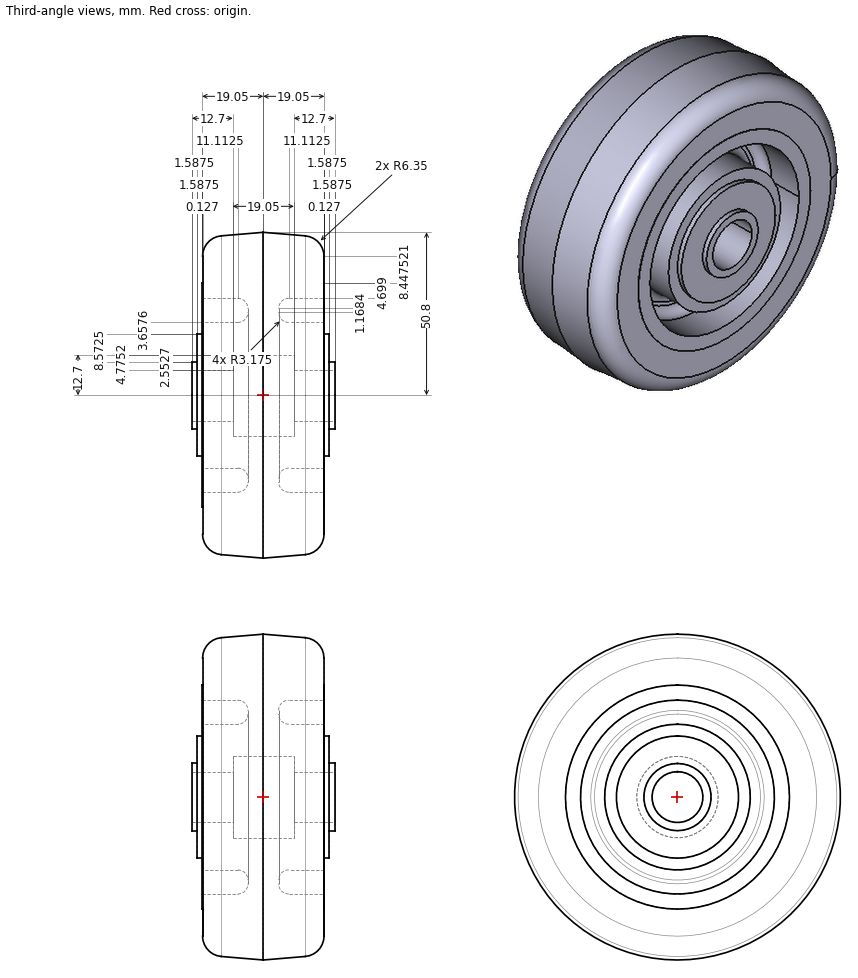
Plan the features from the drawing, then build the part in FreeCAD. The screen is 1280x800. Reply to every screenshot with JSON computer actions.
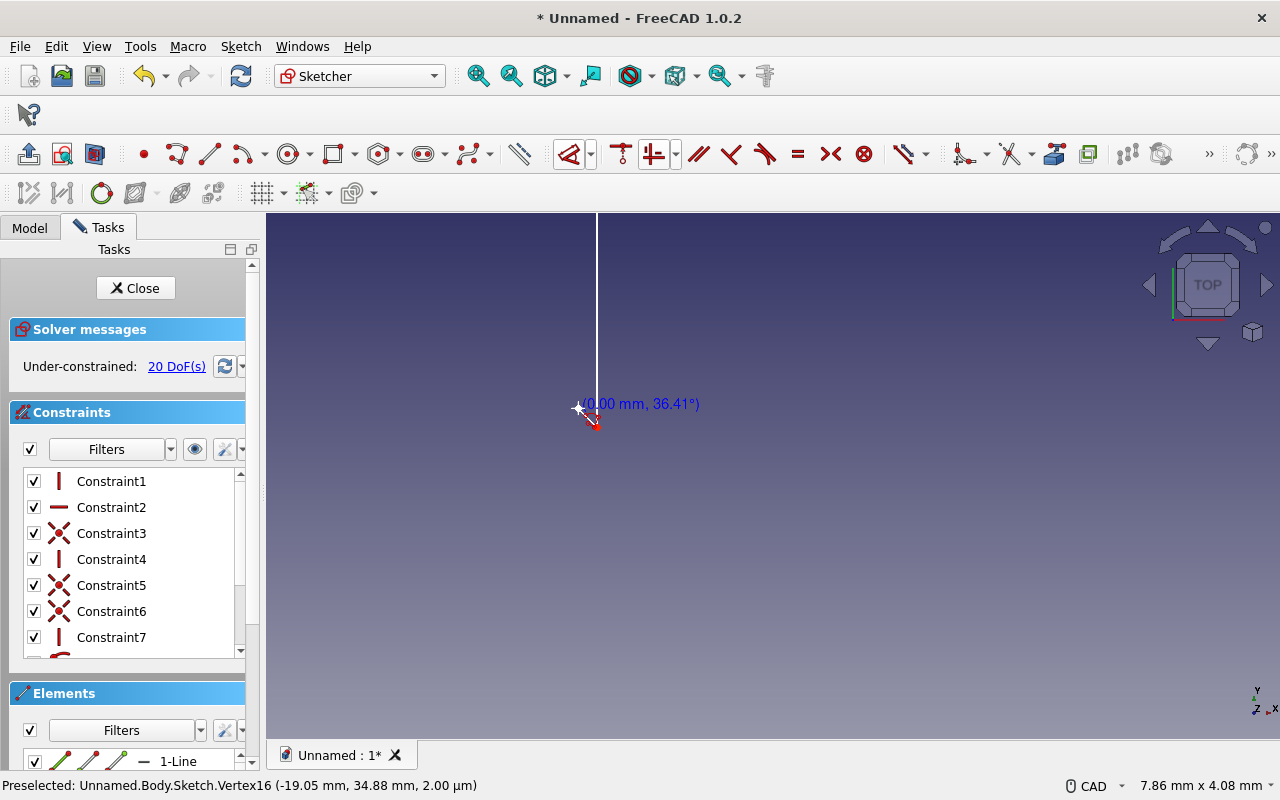
{"action": "scroll", "coordinate": [582, 415], "scroll_direction": "down", "scroll_amount": 15}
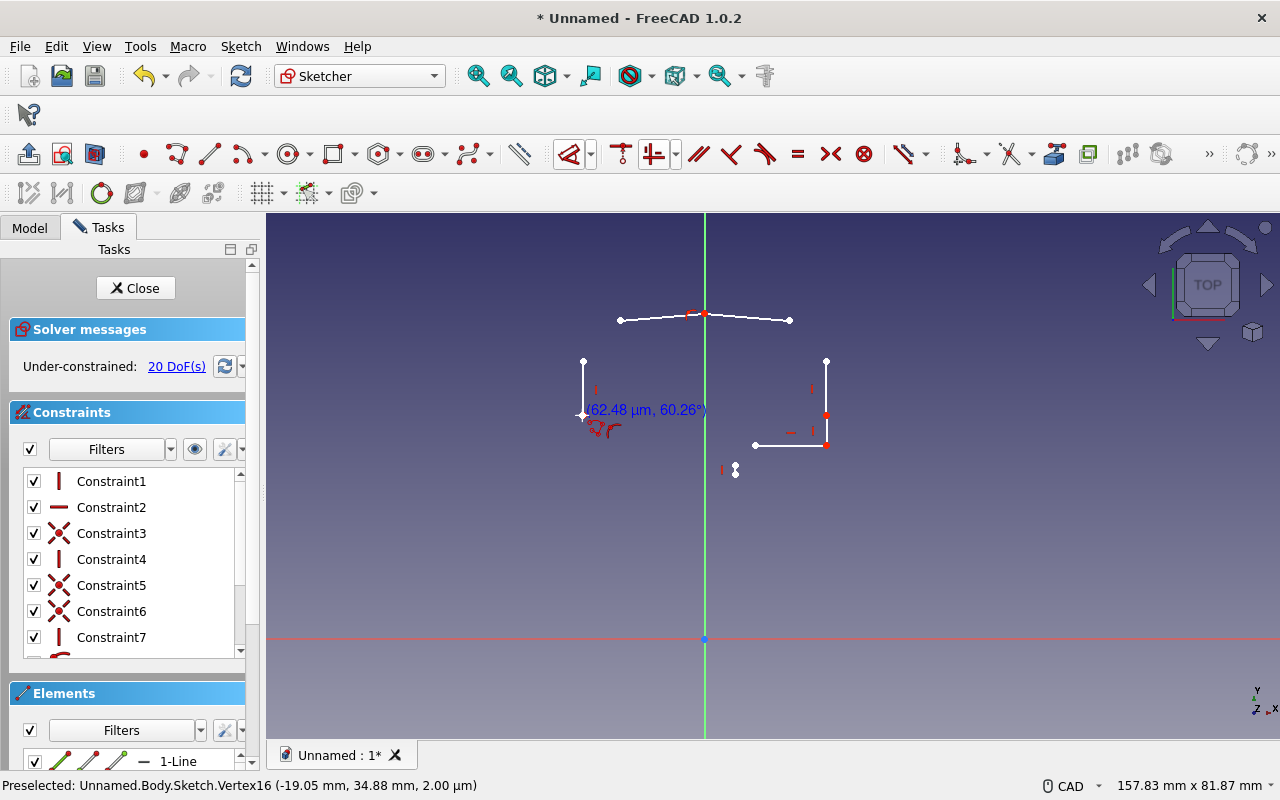
{"action": "left_click", "coordinate": [582, 445]}
{"action": "left_click", "coordinate": [654, 445]}
{"action": "right_click", "coordinate": [654, 445]}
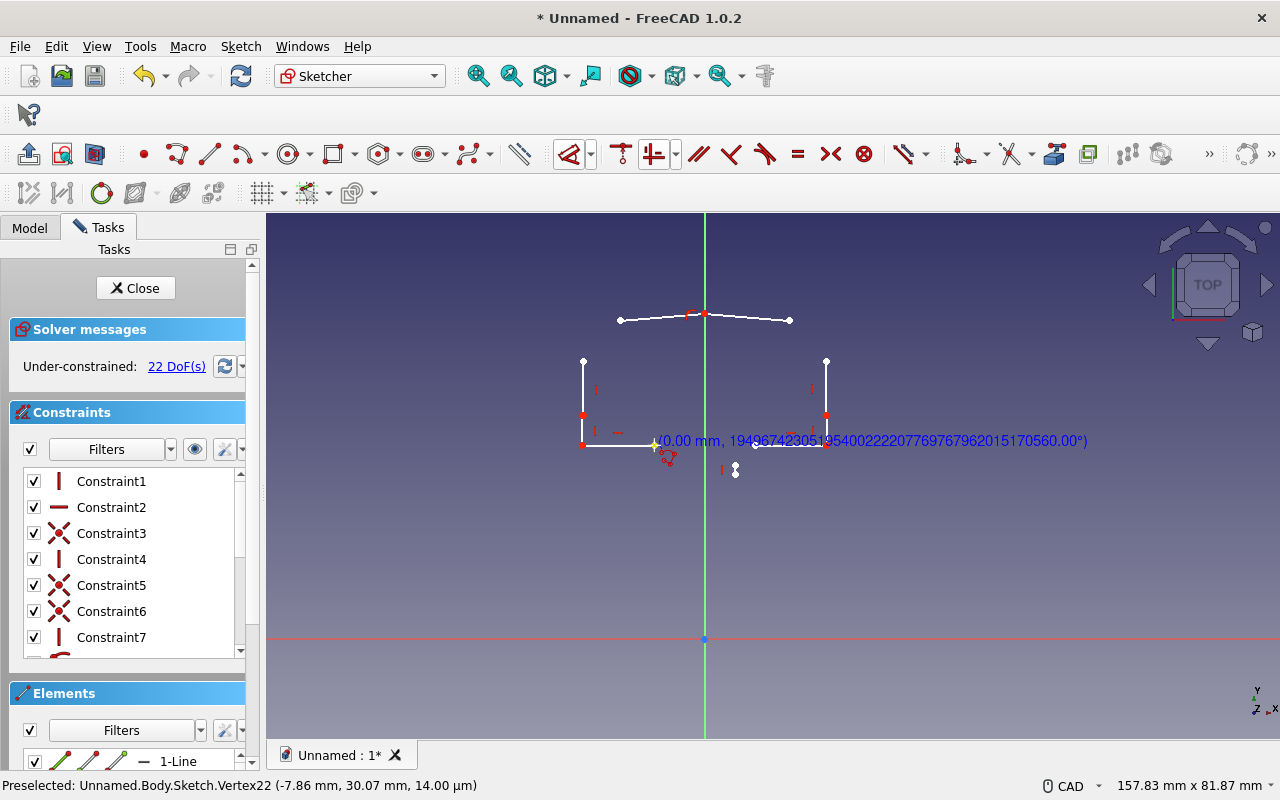
{"action": "left_click", "coordinate": [210, 154]}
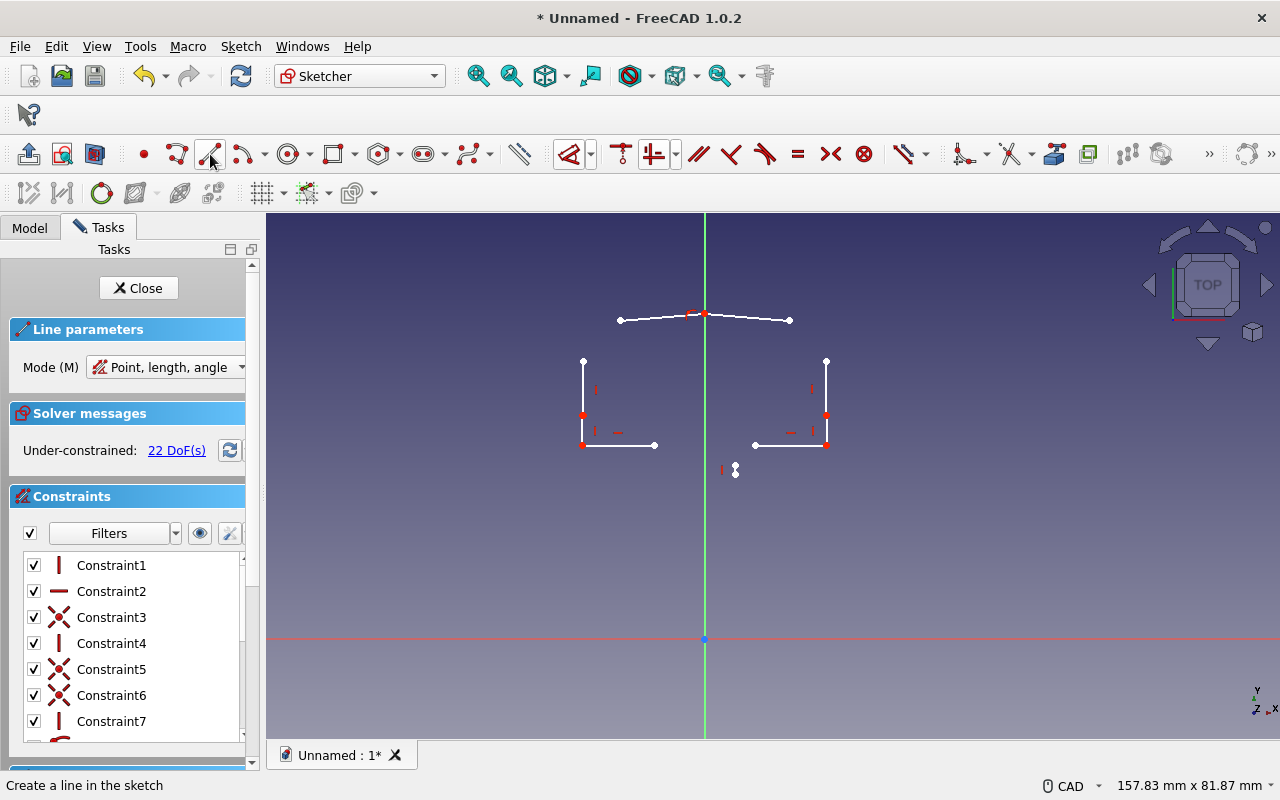
{"action": "left_click", "coordinate": [674, 465]}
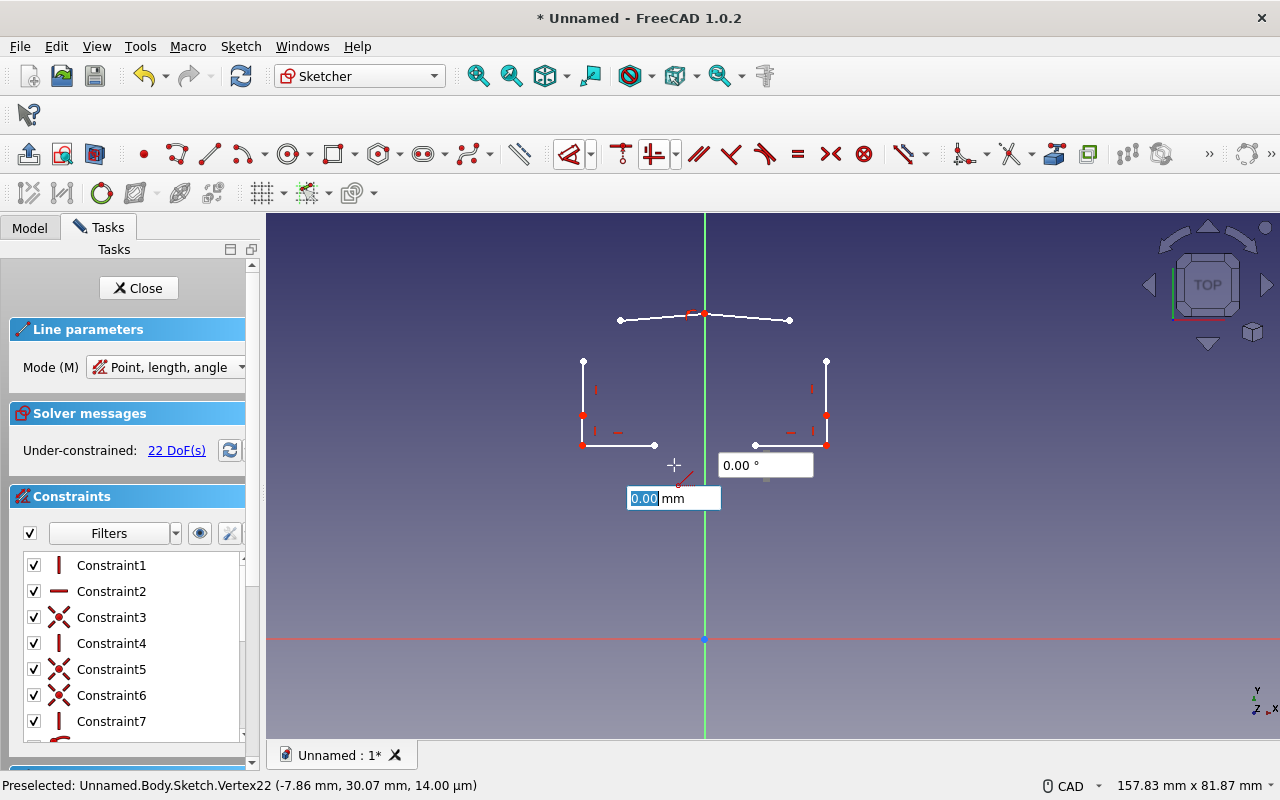
{"action": "scroll", "coordinate": [674, 473], "scroll_direction": "up", "scroll_amount": 4}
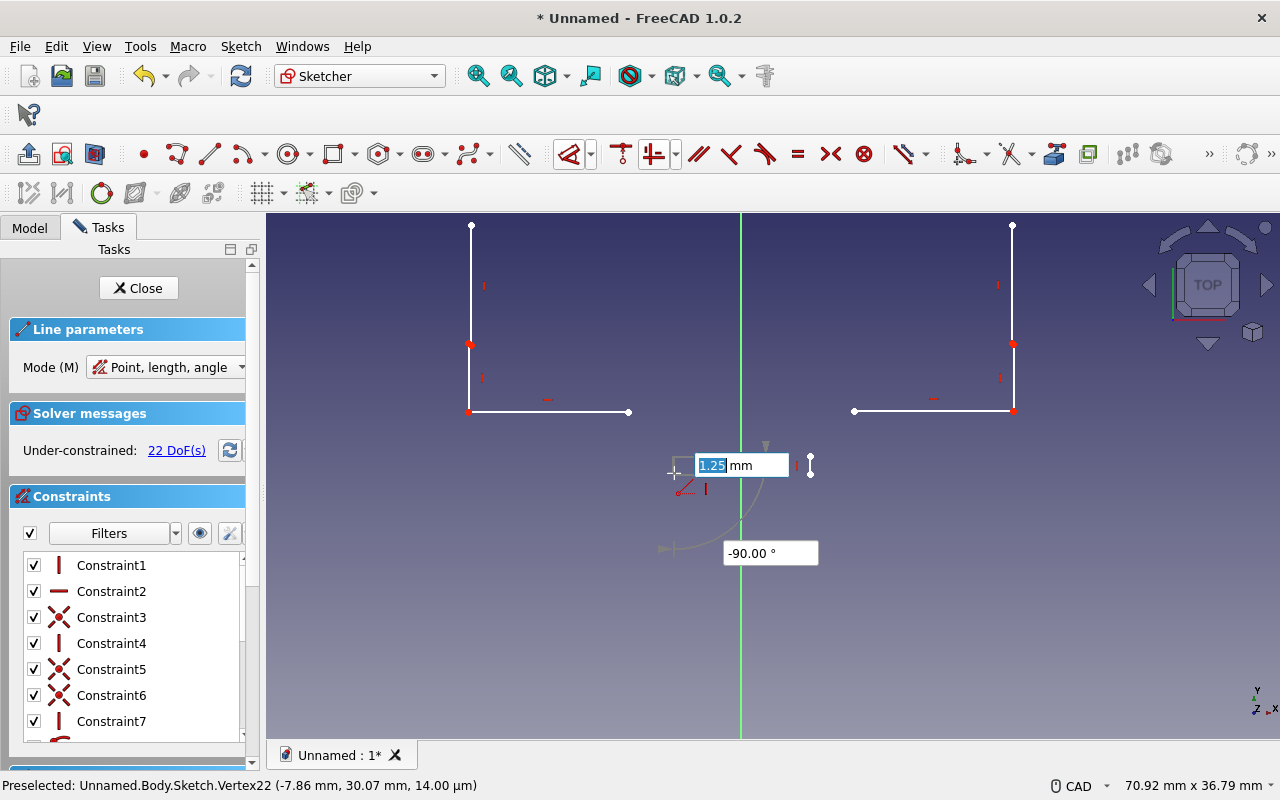
{"action": "left_click", "coordinate": [674, 472]}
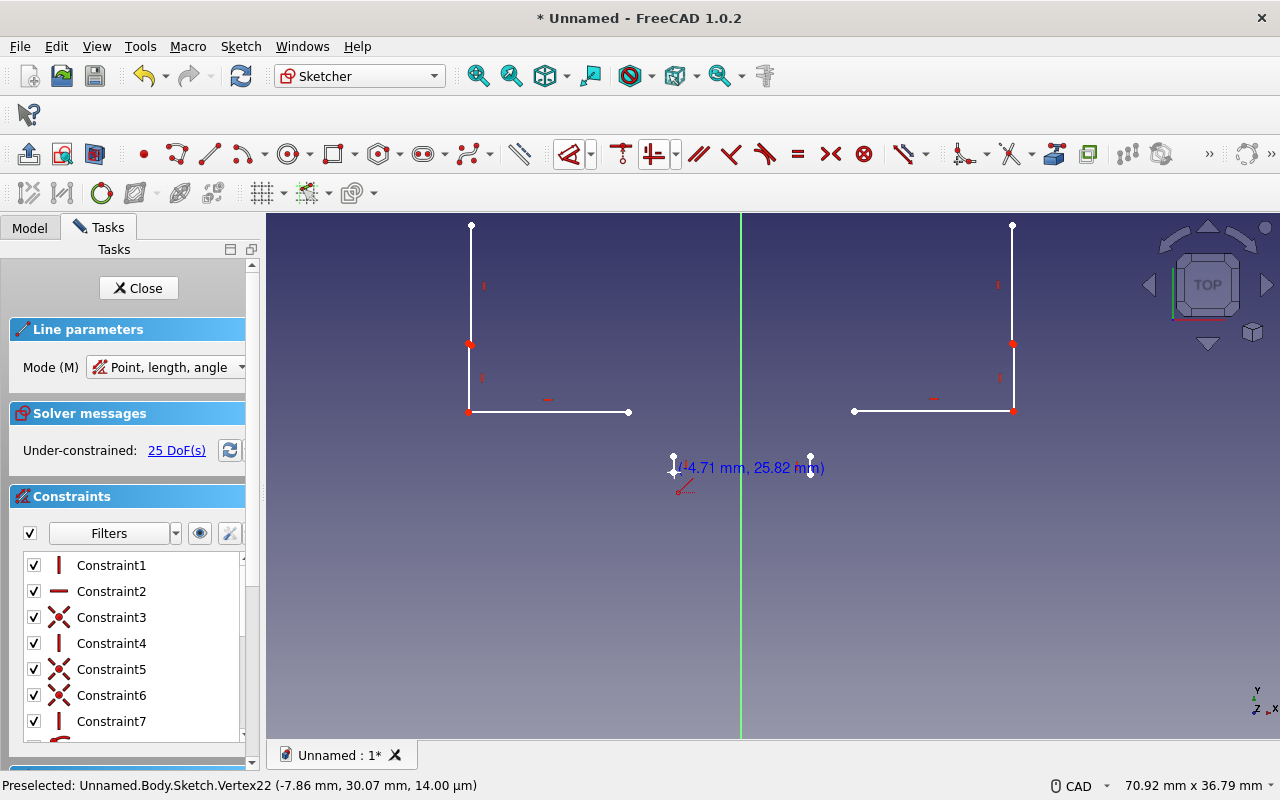
{"action": "left_click", "coordinate": [177, 154]}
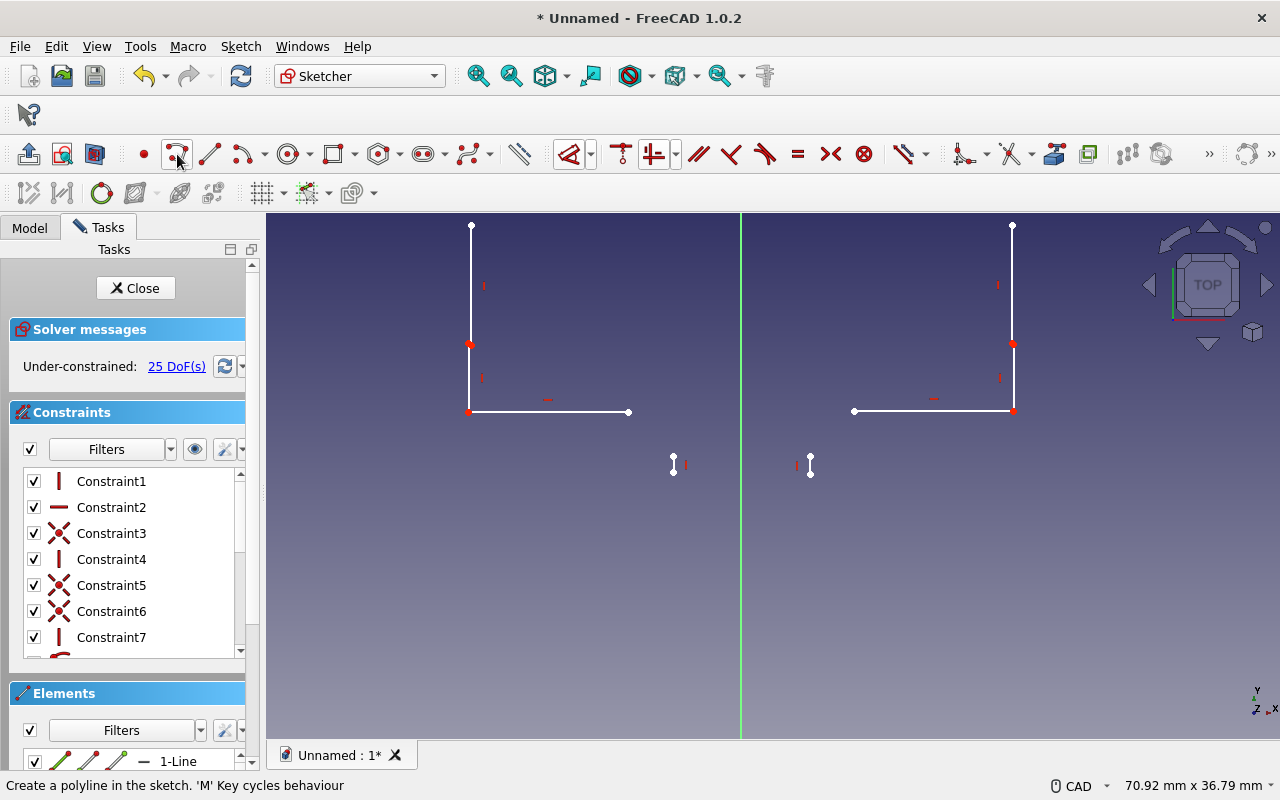
{"action": "left_click", "coordinate": [628, 518]}
{"action": "left_click", "coordinate": [469, 518]}
{"action": "left_click", "coordinate": [469, 570]}
{"action": "left_click", "coordinate": [446, 570]}
{"action": "left_click", "coordinate": [446, 692]}
{"action": "left_click", "coordinate": [424, 692]}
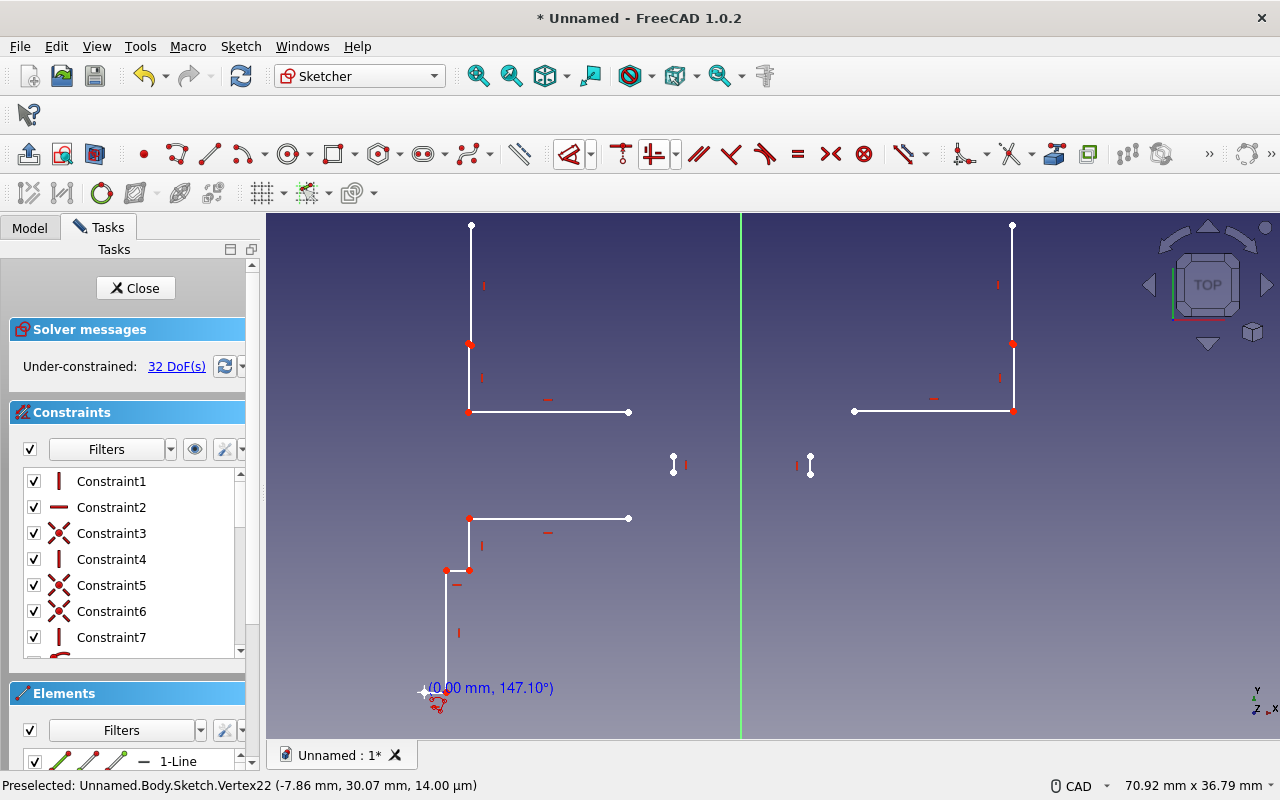
{"action": "scroll", "coordinate": [674, 473], "scroll_direction": "down", "scroll_amount": 4}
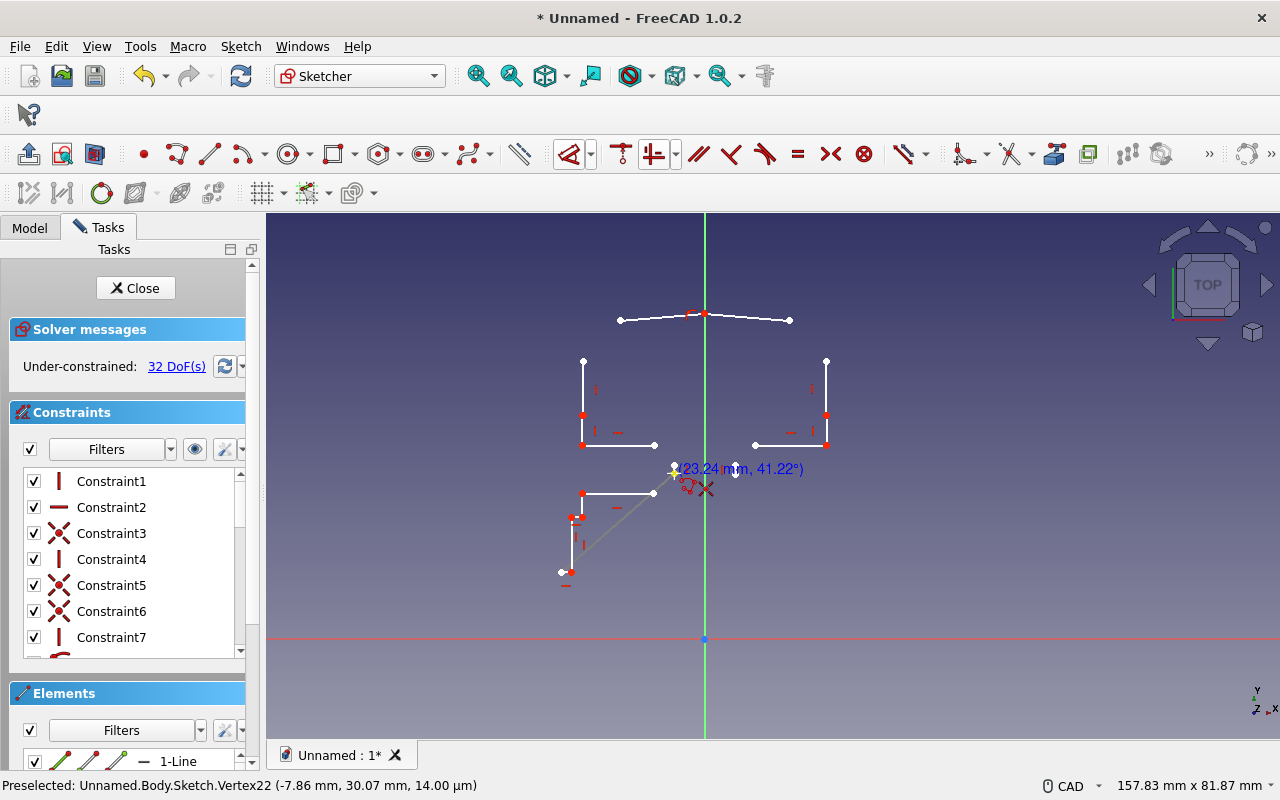
{"action": "left_click", "coordinate": [562, 588]}
{"action": "left_click", "coordinate": [643, 588]}
{"action": "left_click", "coordinate": [643, 558]}
{"action": "left_click", "coordinate": [766, 558]}
{"action": "left_click", "coordinate": [766, 588]}
{"action": "left_click", "coordinate": [847, 588]}
{"action": "left_click", "coordinate": [847, 572]}